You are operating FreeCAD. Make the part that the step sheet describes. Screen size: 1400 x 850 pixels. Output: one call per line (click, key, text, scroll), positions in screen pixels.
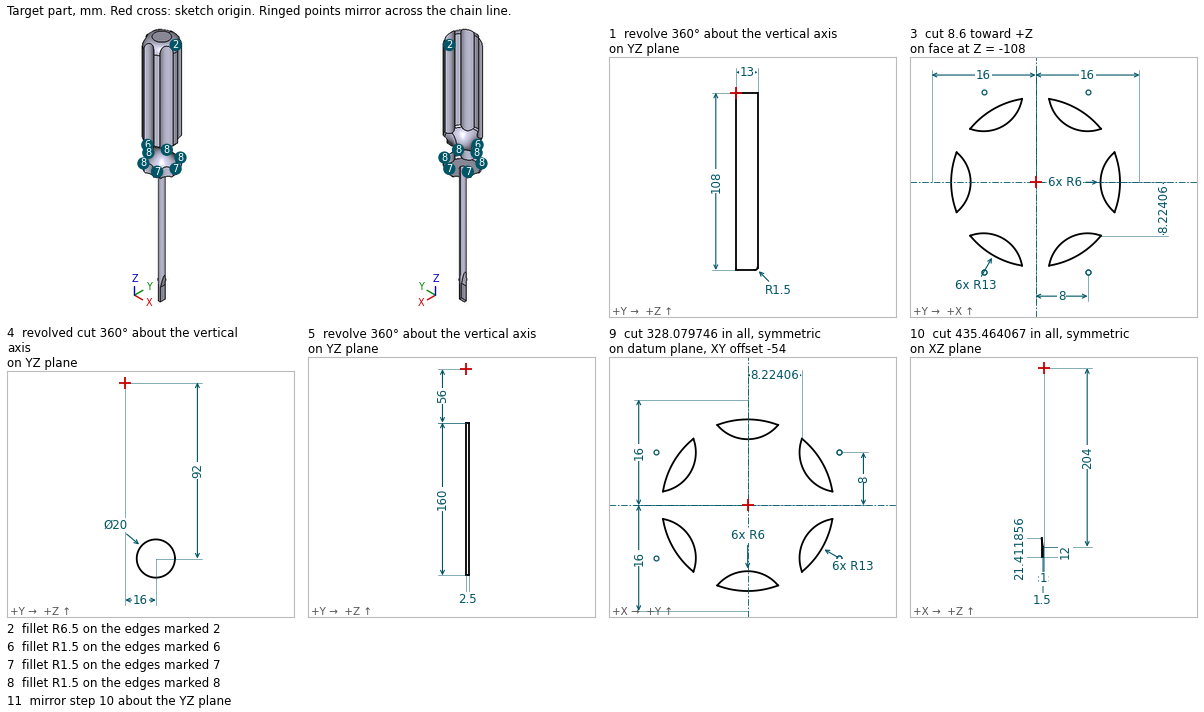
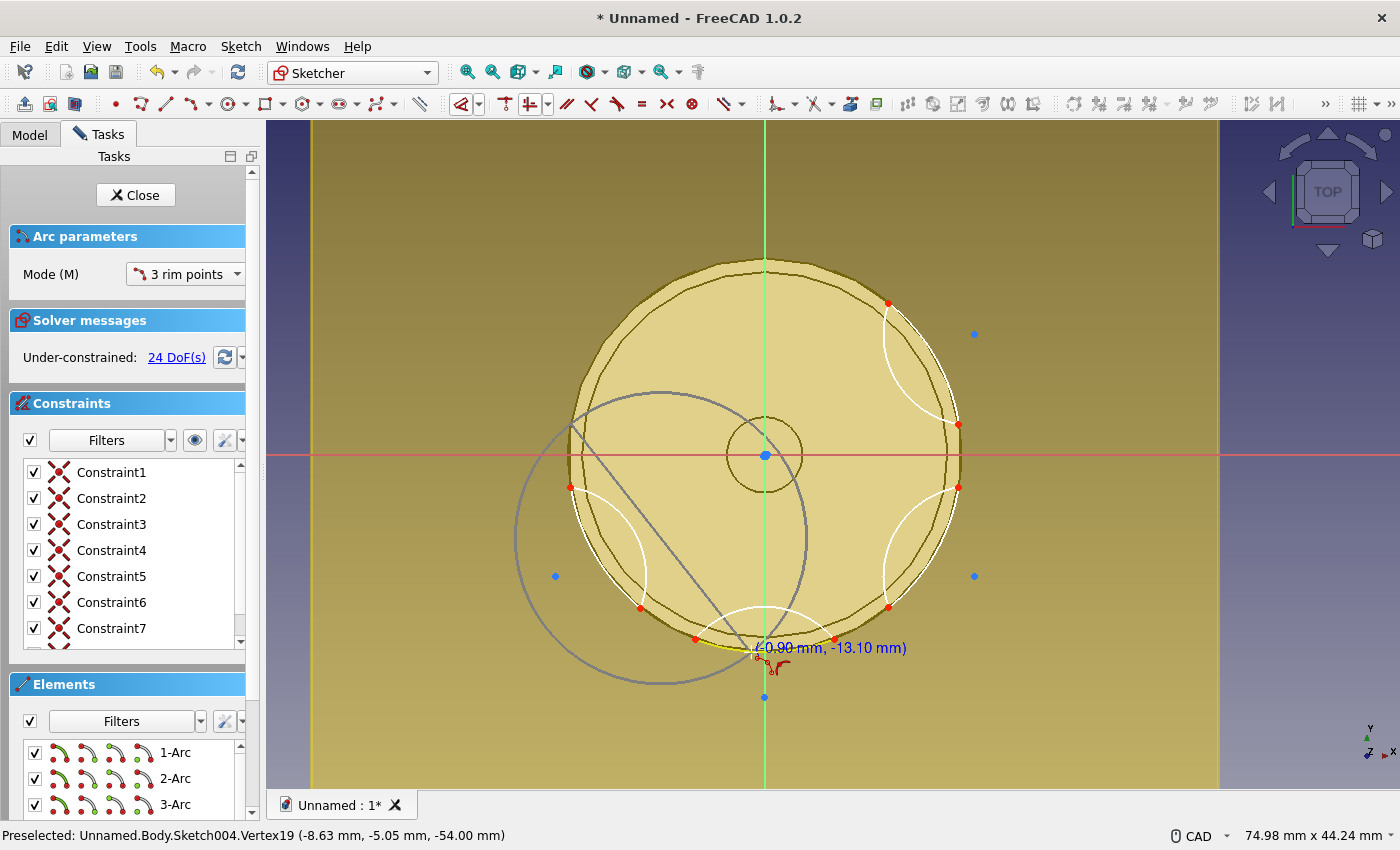
click(640, 303)
click(634, 379)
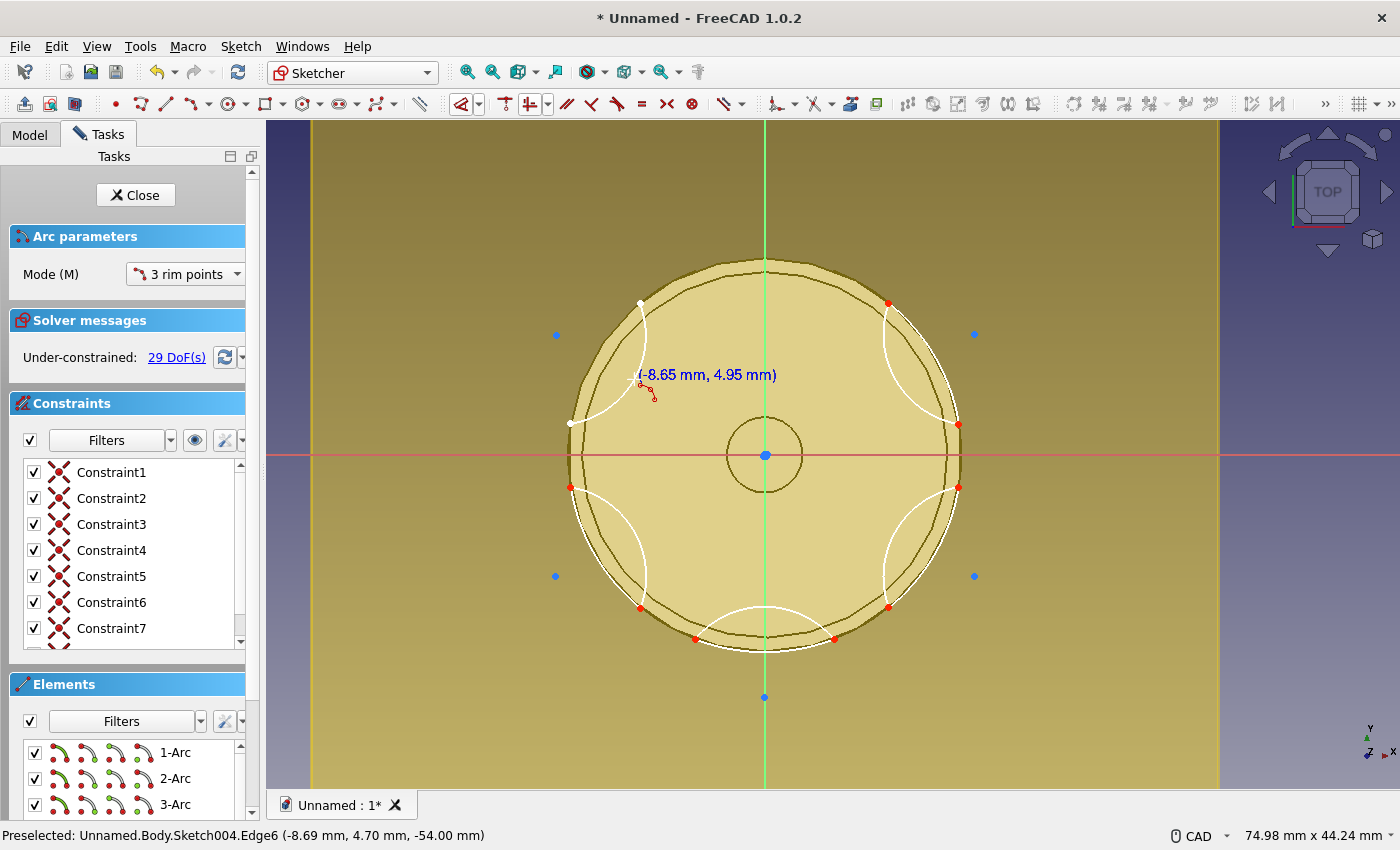
click(640, 304)
click(571, 424)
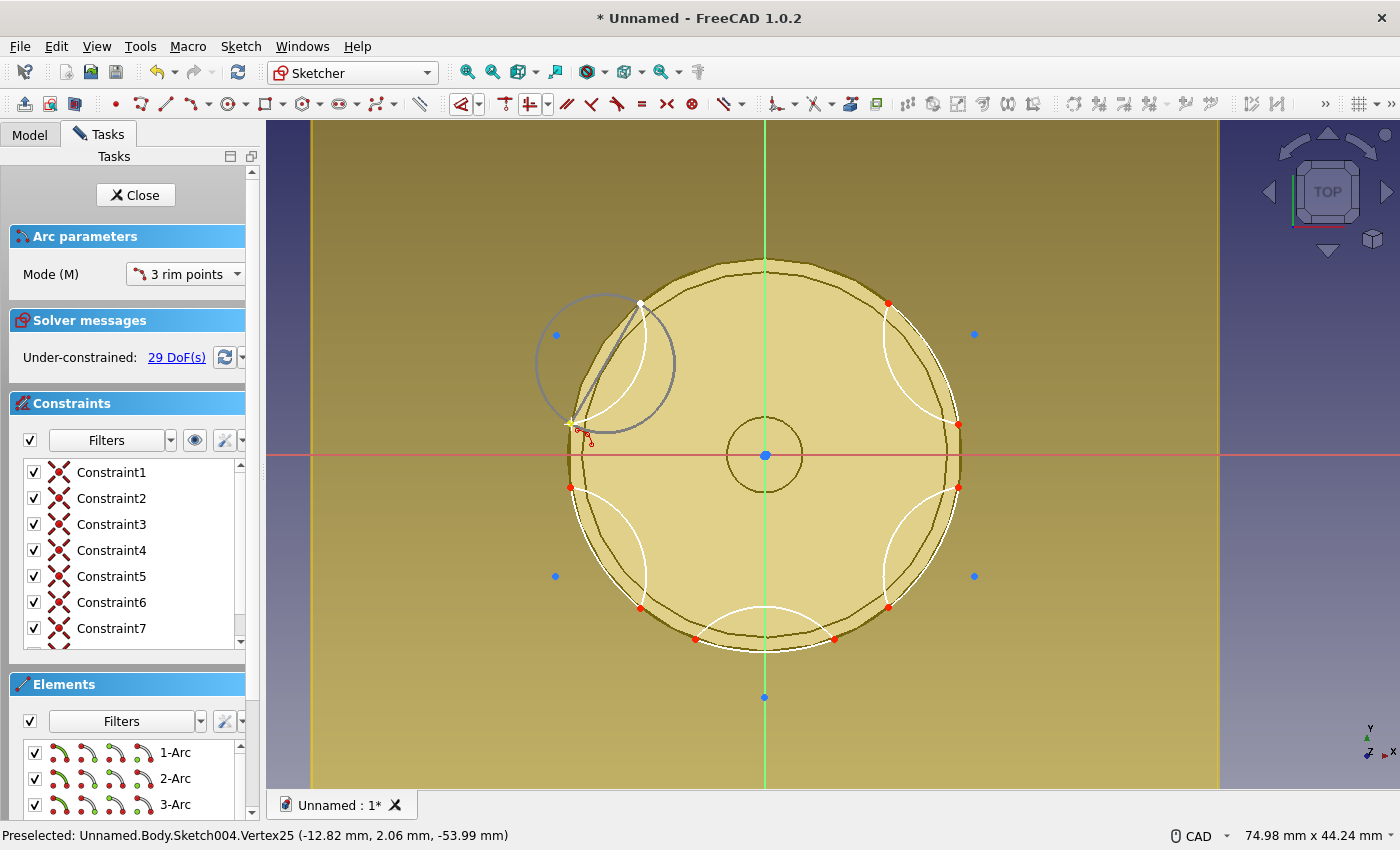
scroll(594, 357, up, 2)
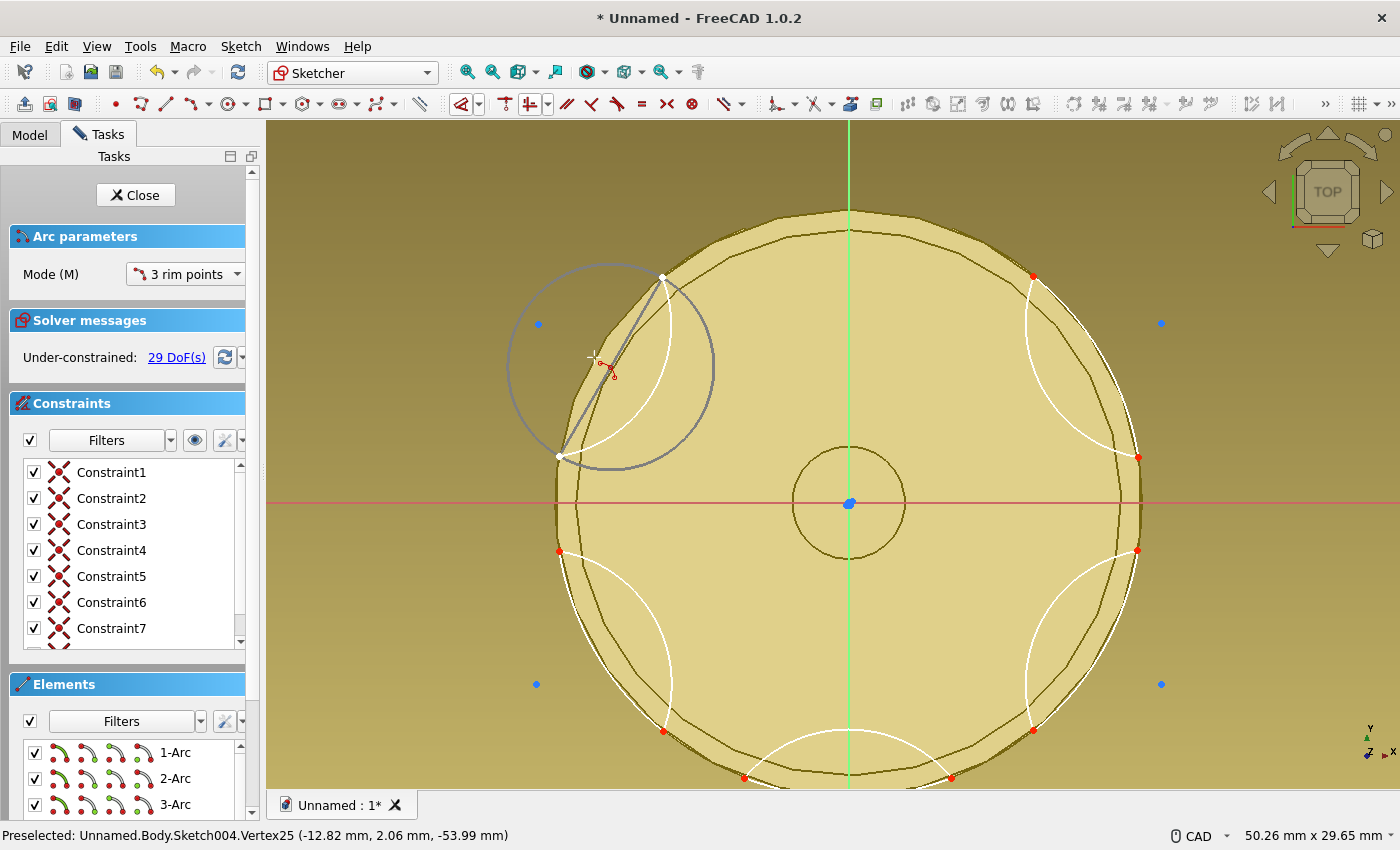
click(595, 356)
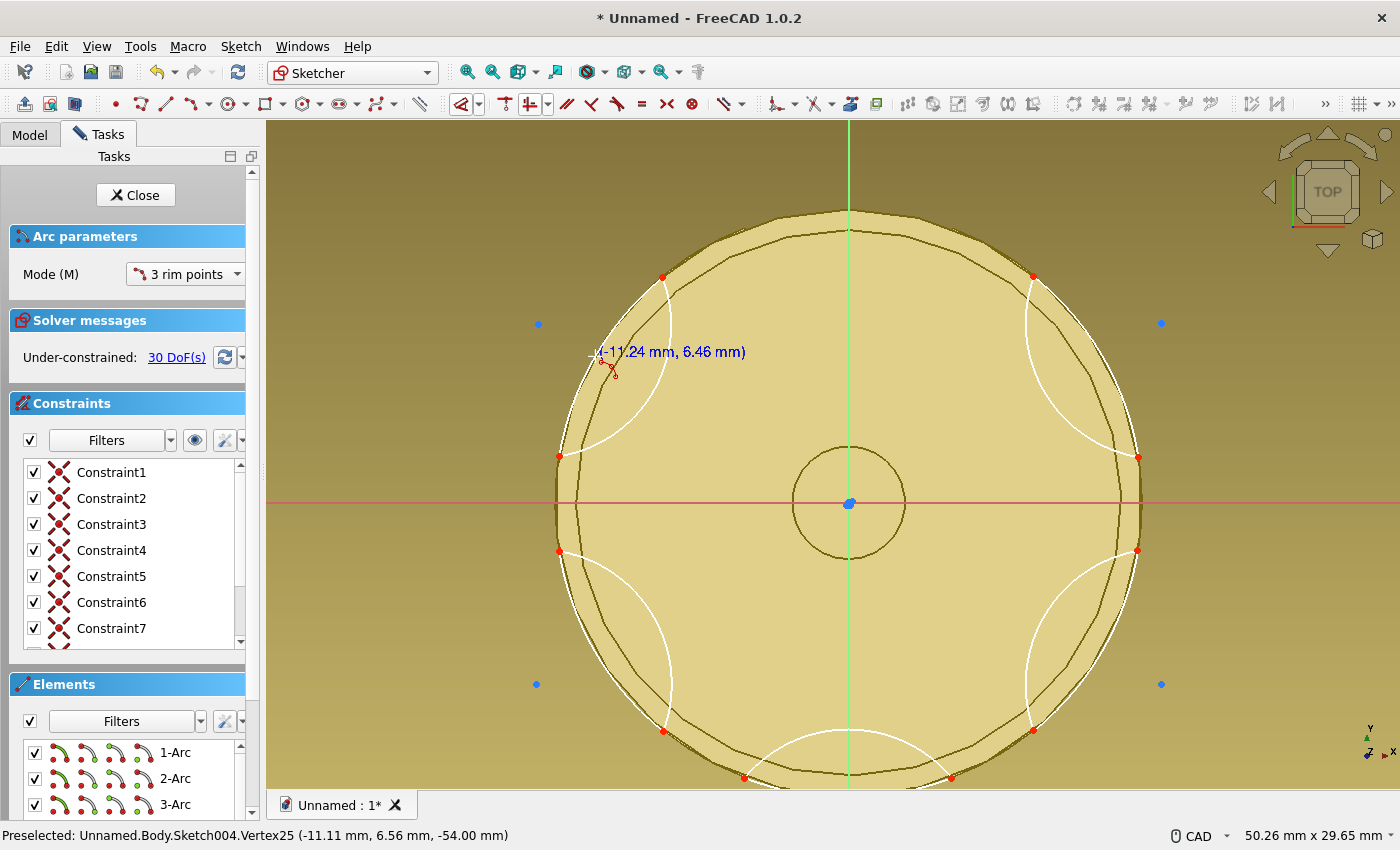
click(745, 229)
click(953, 229)
click(825, 275)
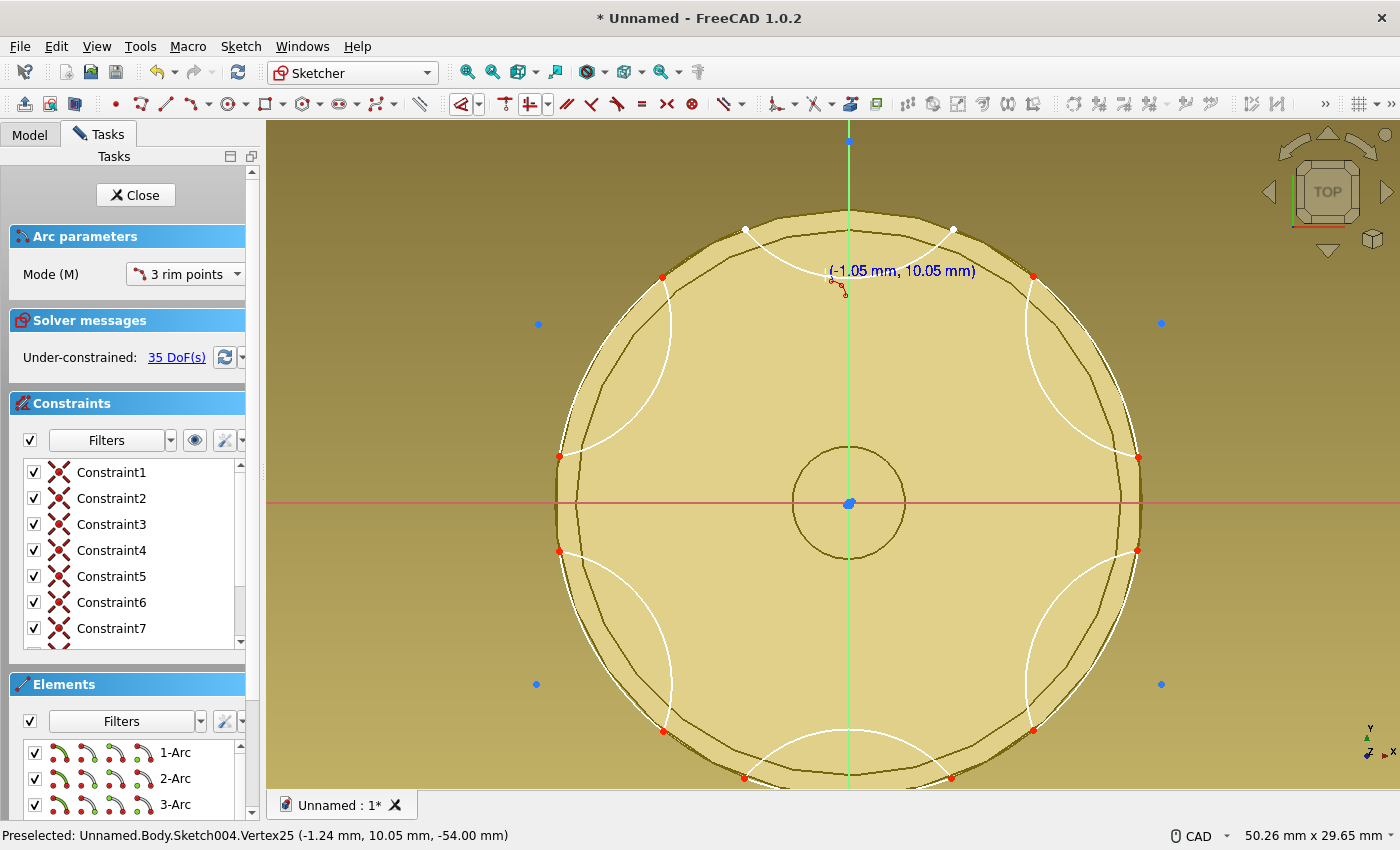
click(953, 230)
click(745, 230)
click(870, 210)
key(Escape)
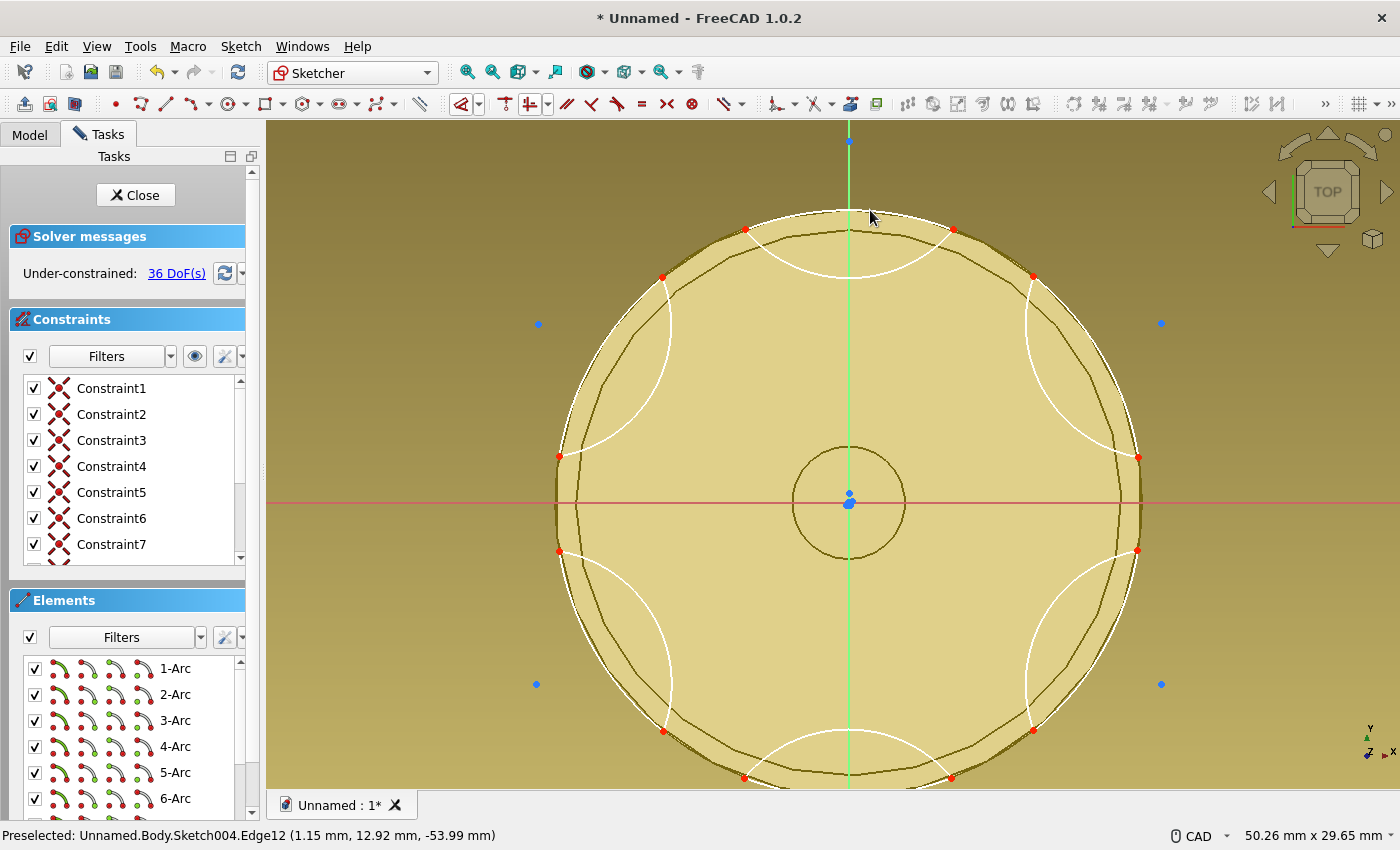
click(1122, 396)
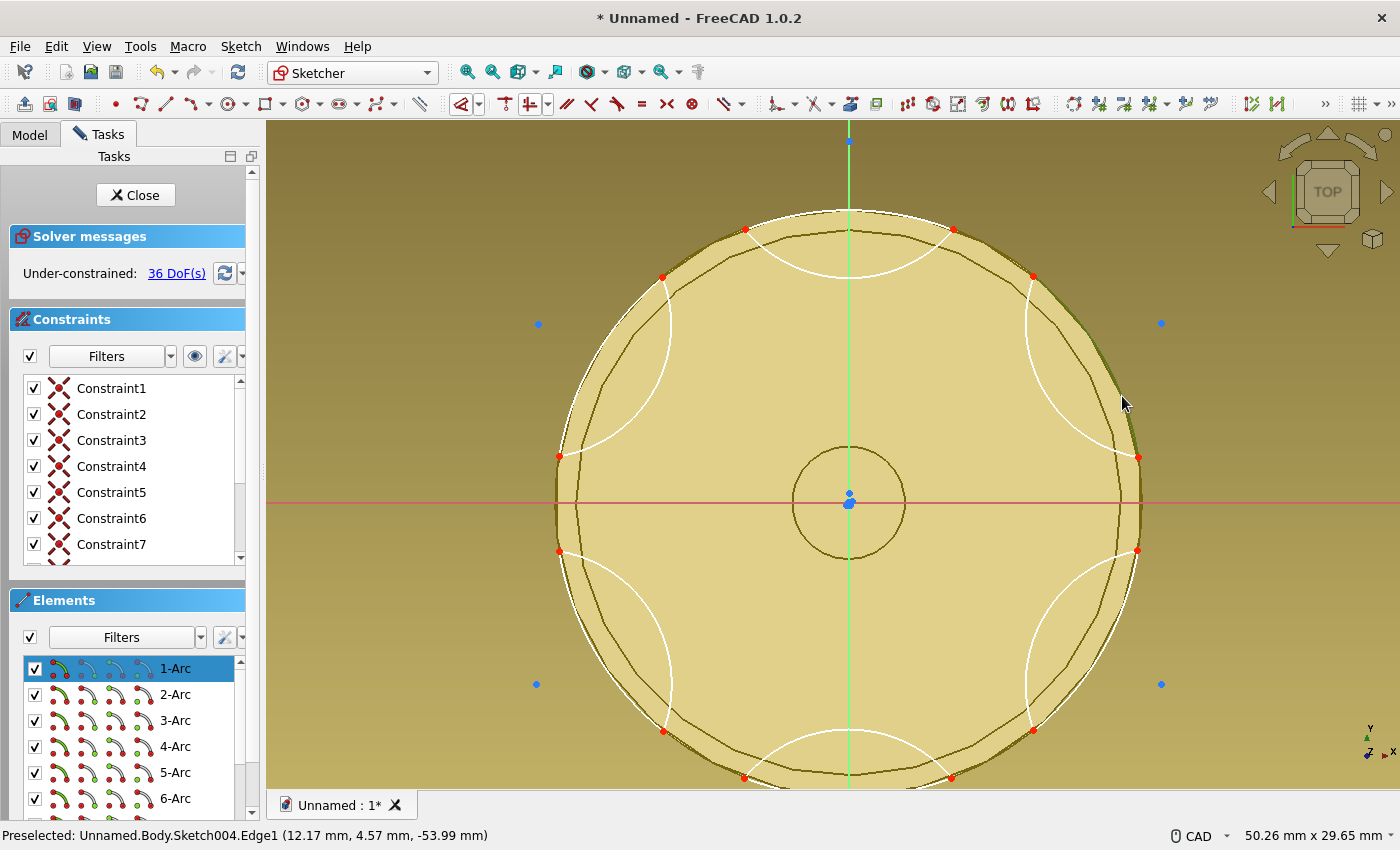
click(1079, 686)